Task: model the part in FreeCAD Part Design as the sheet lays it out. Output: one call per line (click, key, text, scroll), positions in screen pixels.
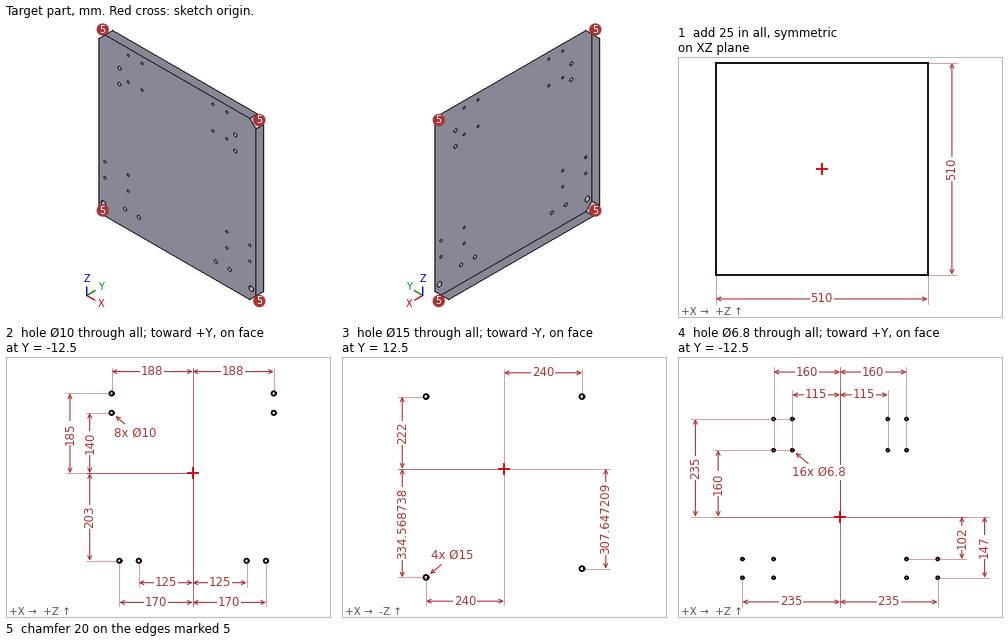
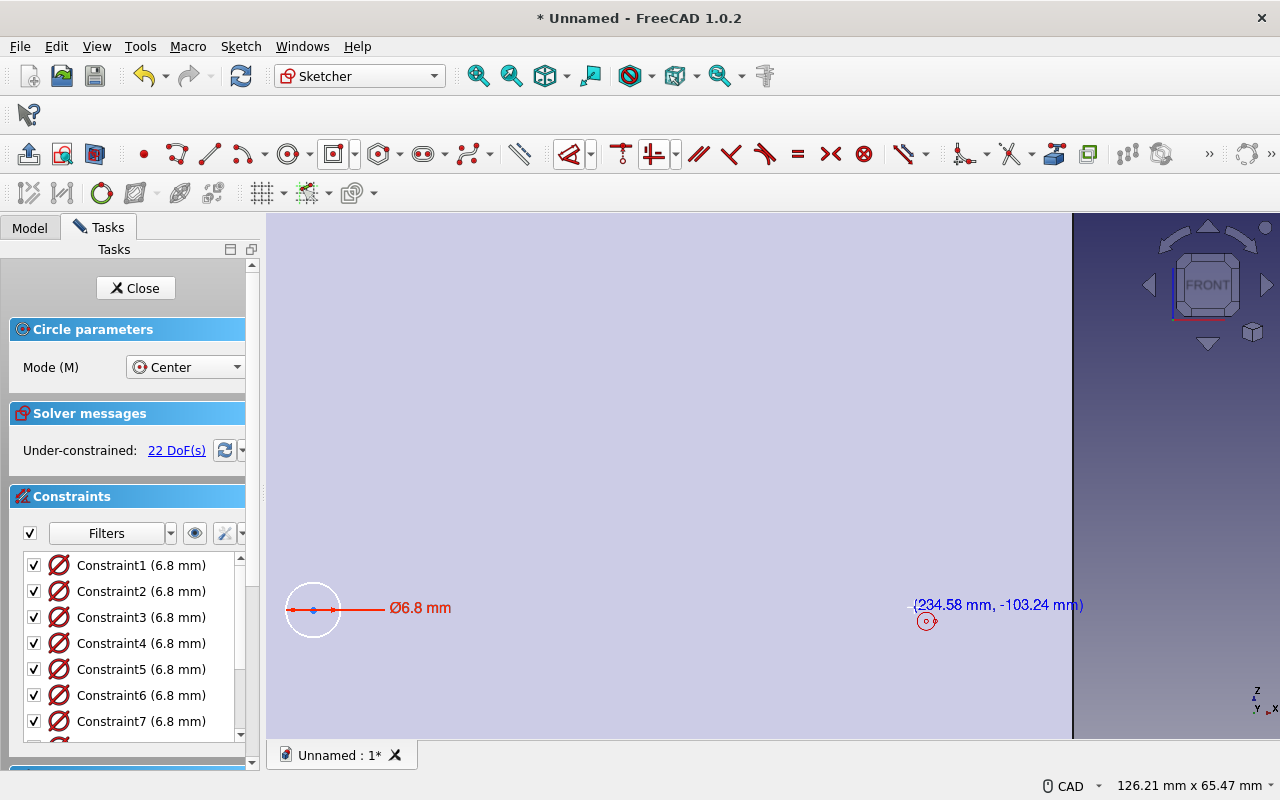
scroll(914, 607, down, 11)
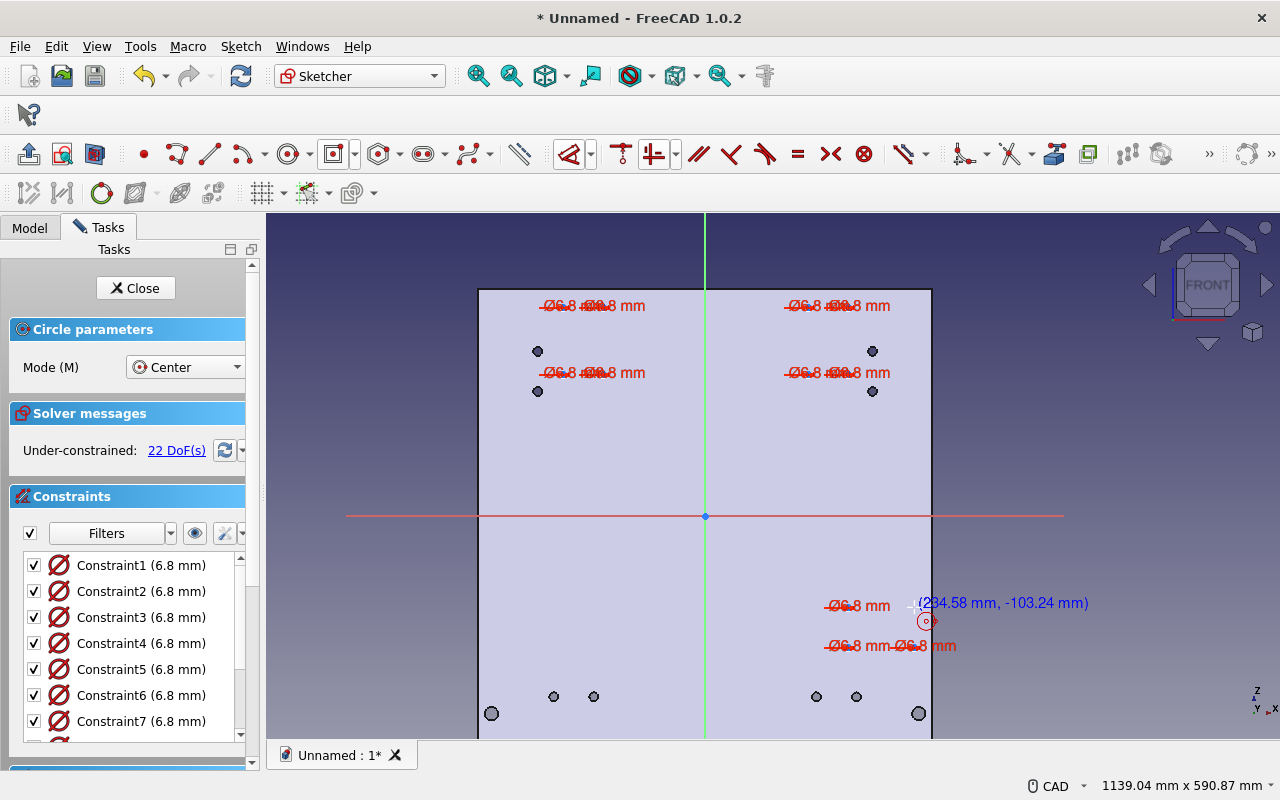
click(914, 607)
move(917, 605)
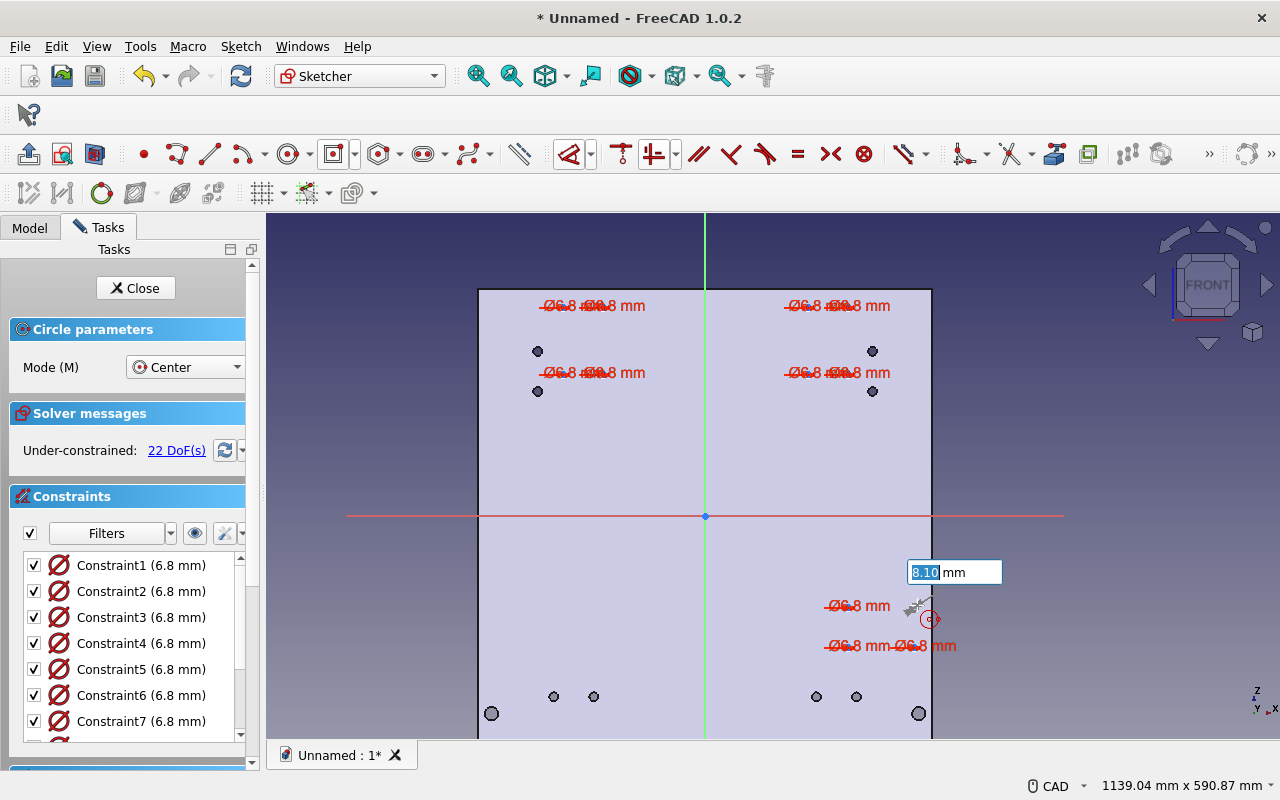
text(6.8)
key(Return)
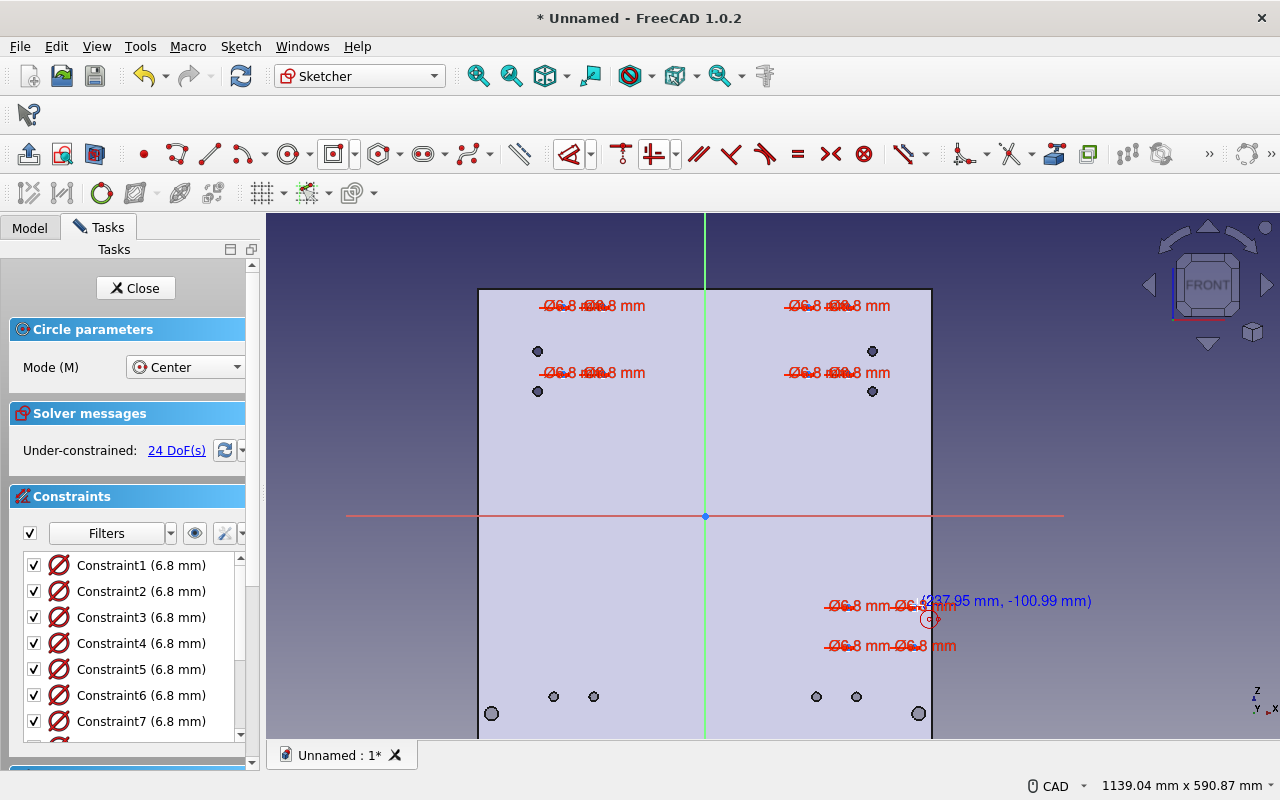
scroll(563, 647, up, 11)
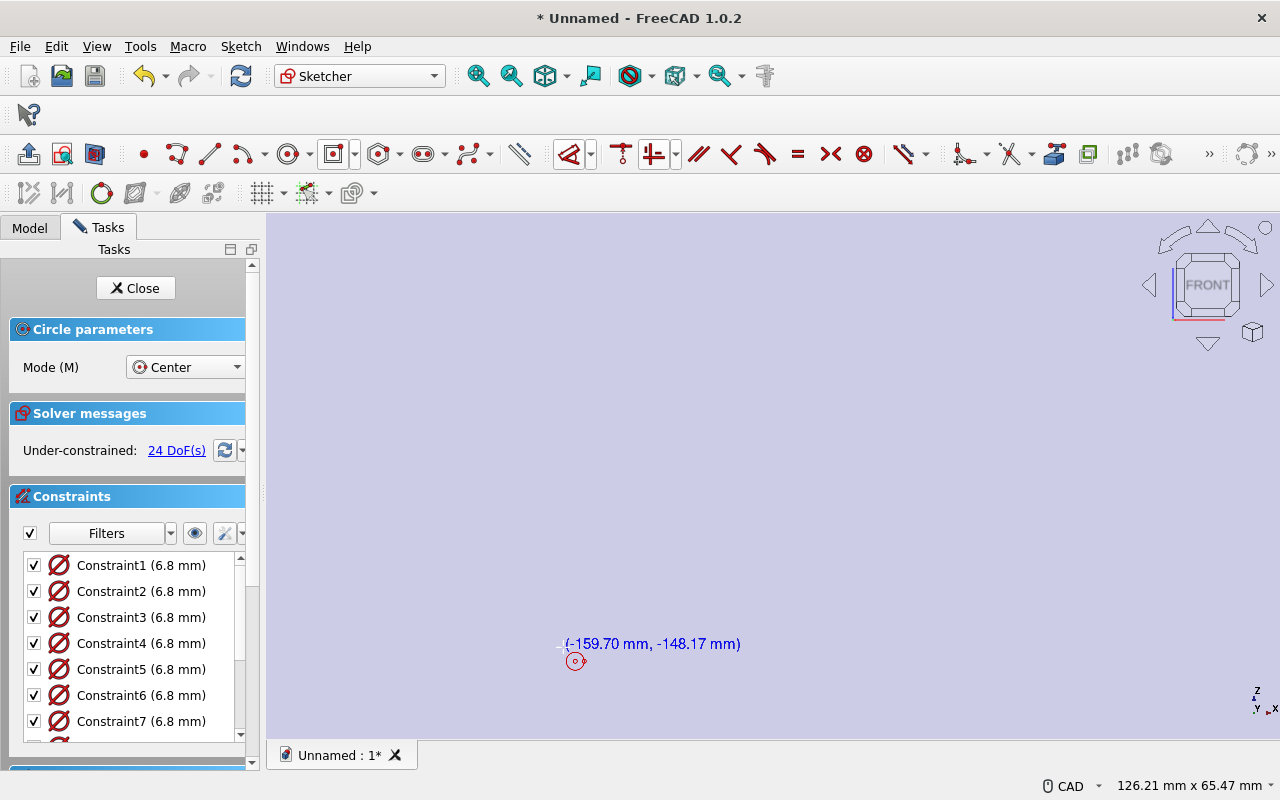
scroll(563, 647, down, 11)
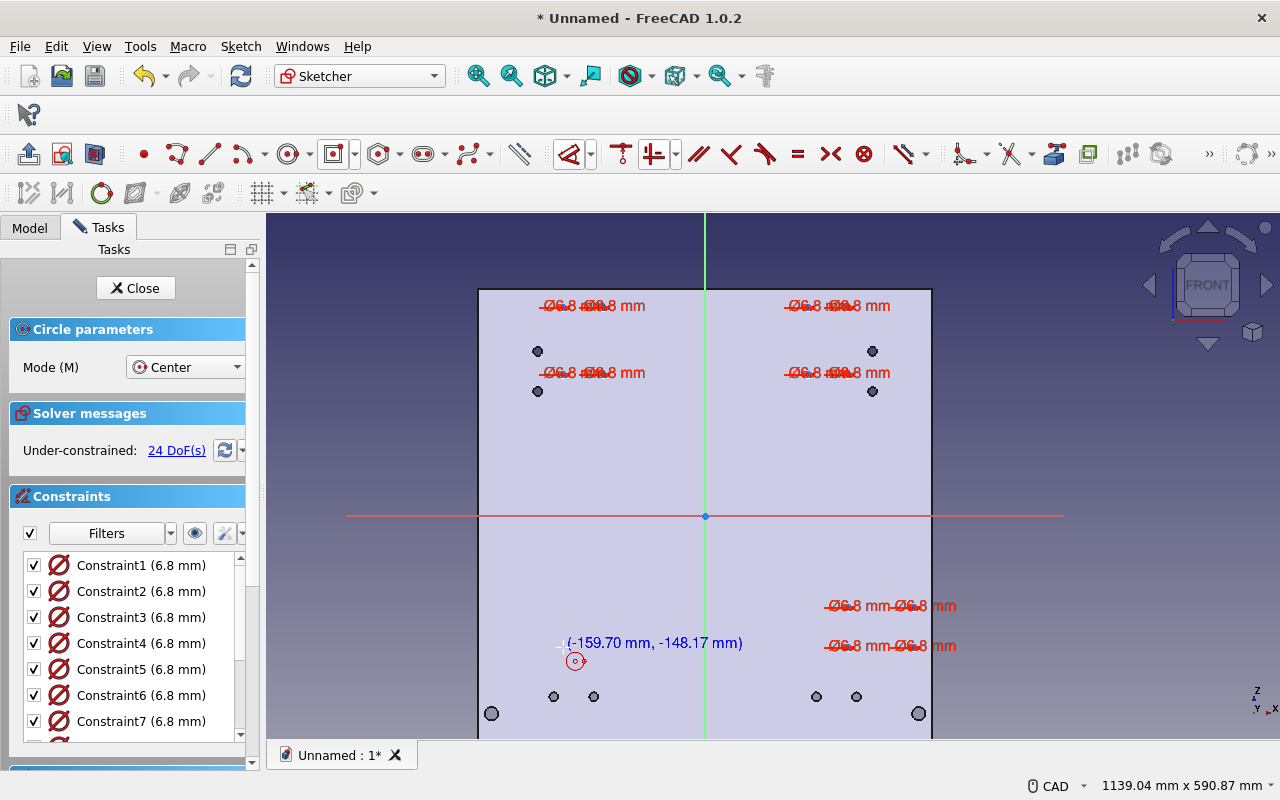
click(563, 647)
move(565, 645)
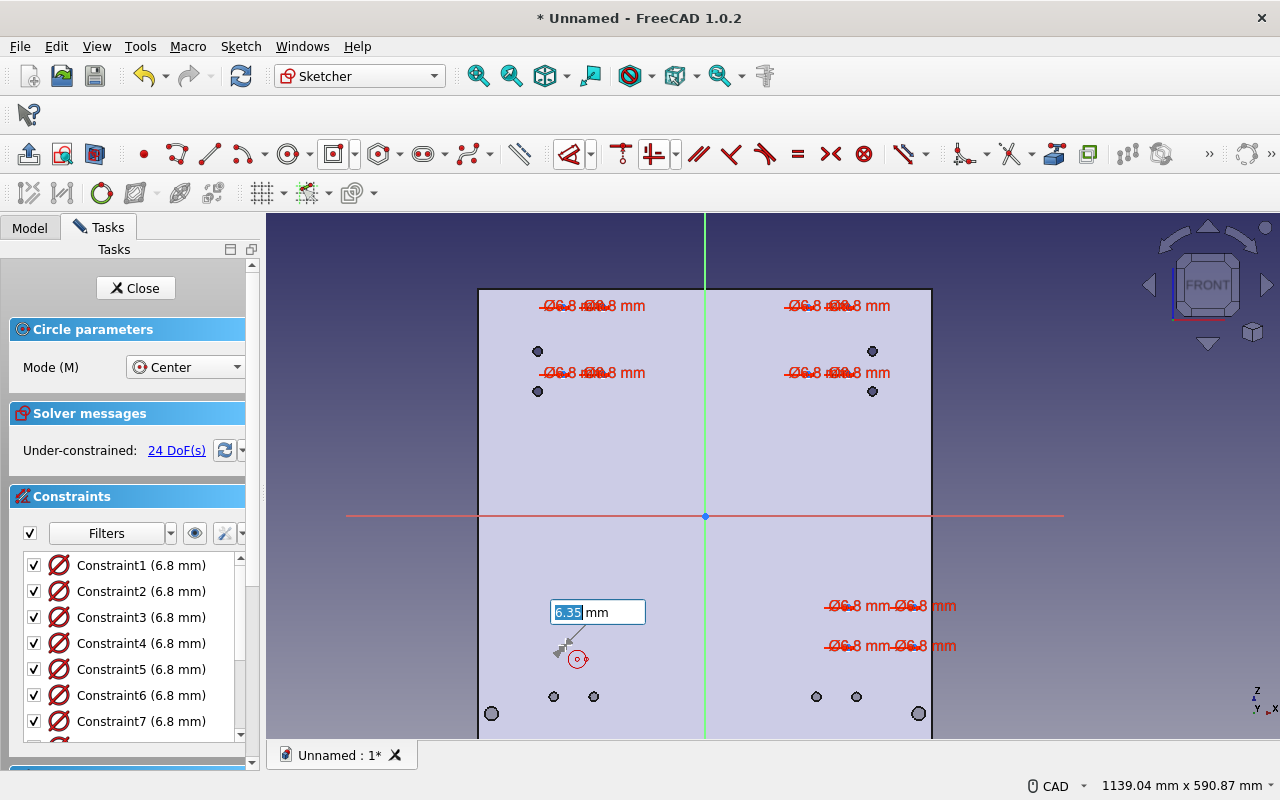
text(6.8)
key(Return)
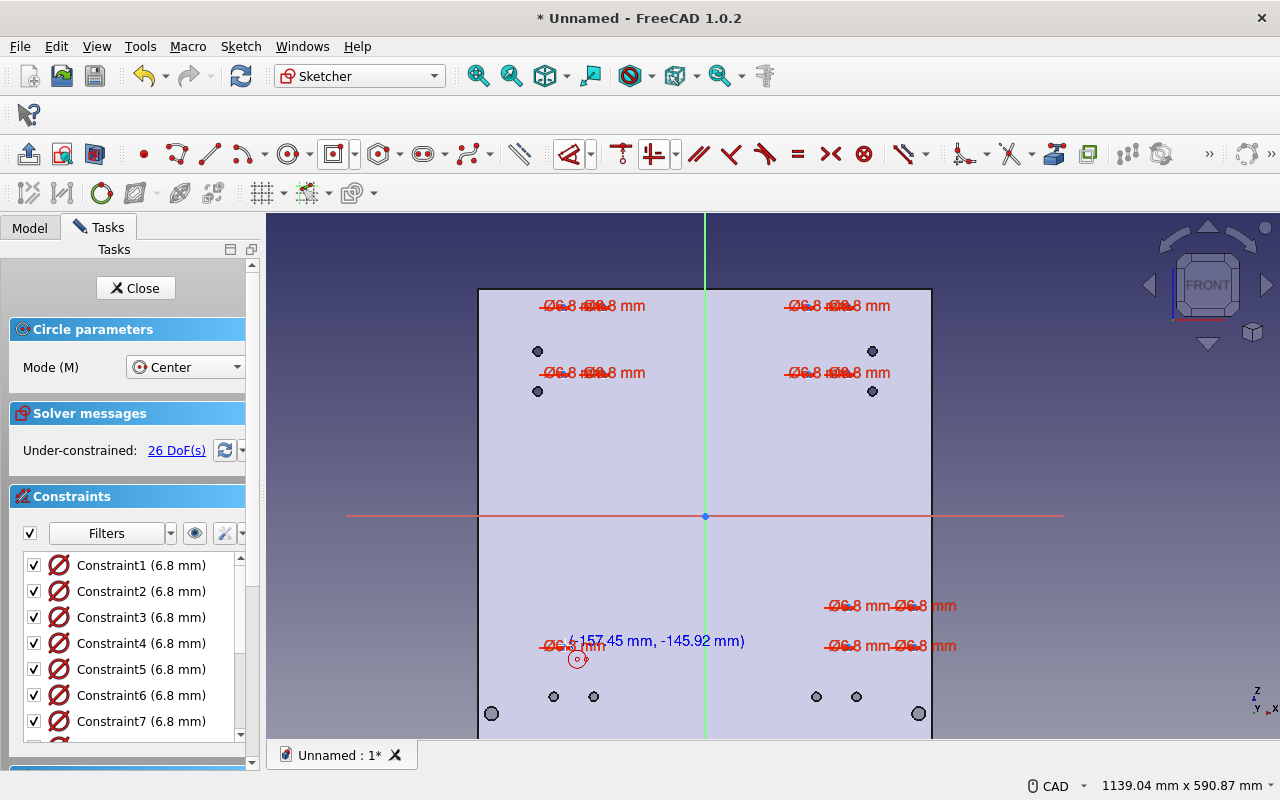
scroll(496, 647, up, 11)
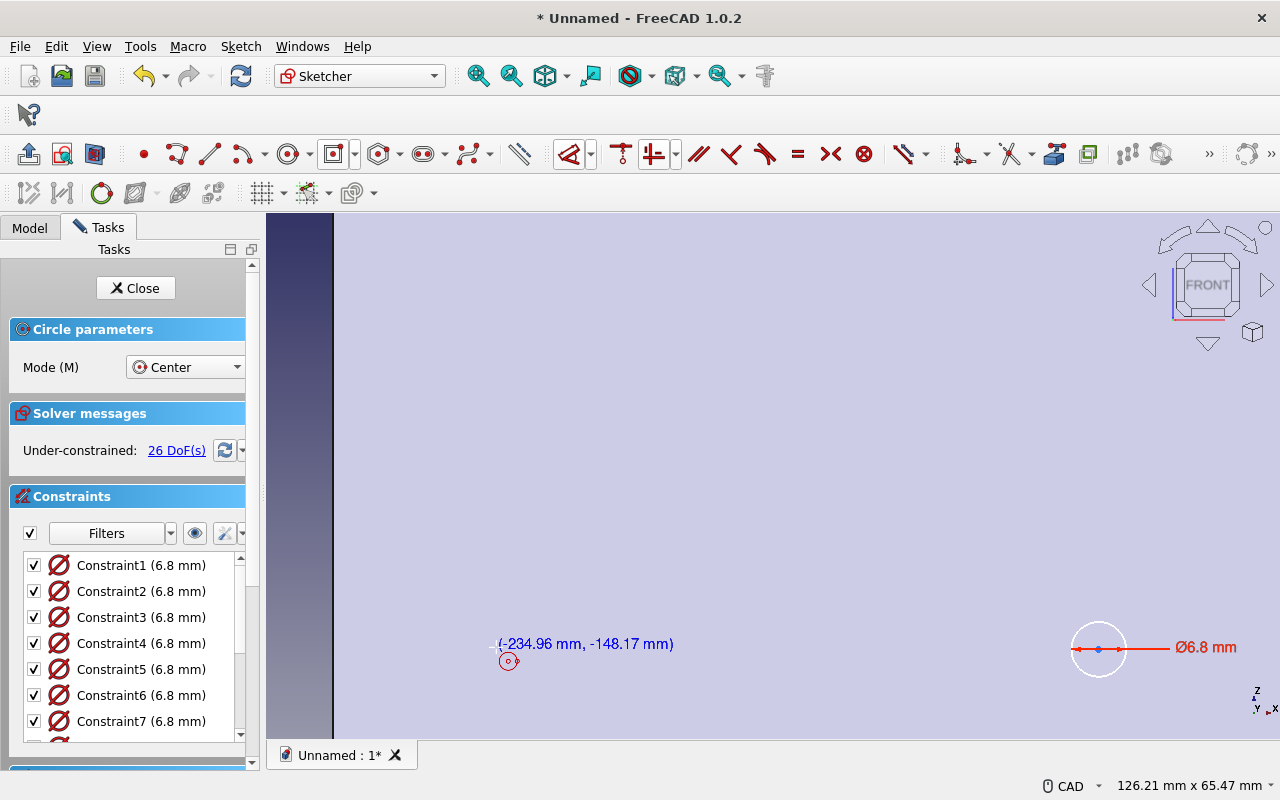
scroll(495, 647, down, 11)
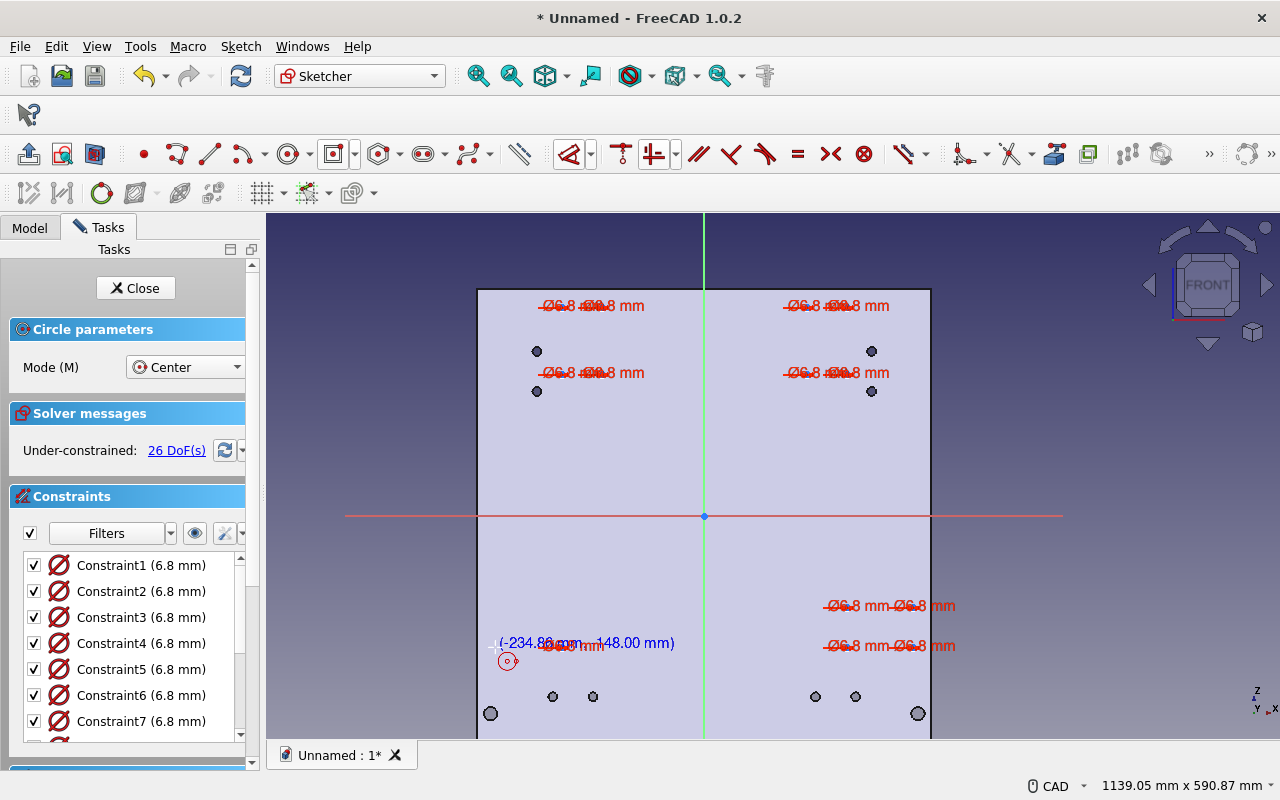
click(495, 647)
move(497, 645)